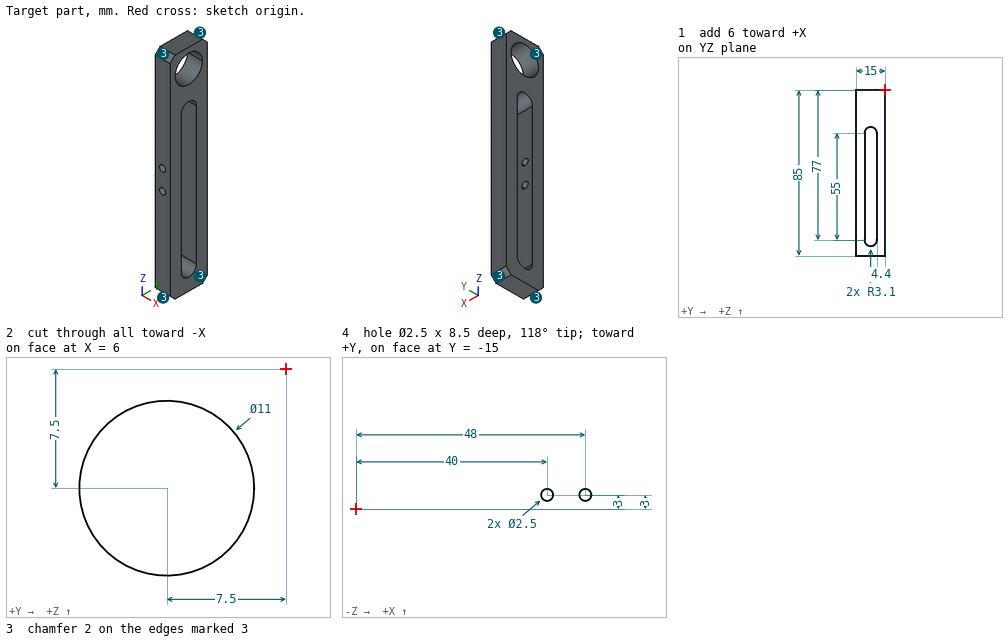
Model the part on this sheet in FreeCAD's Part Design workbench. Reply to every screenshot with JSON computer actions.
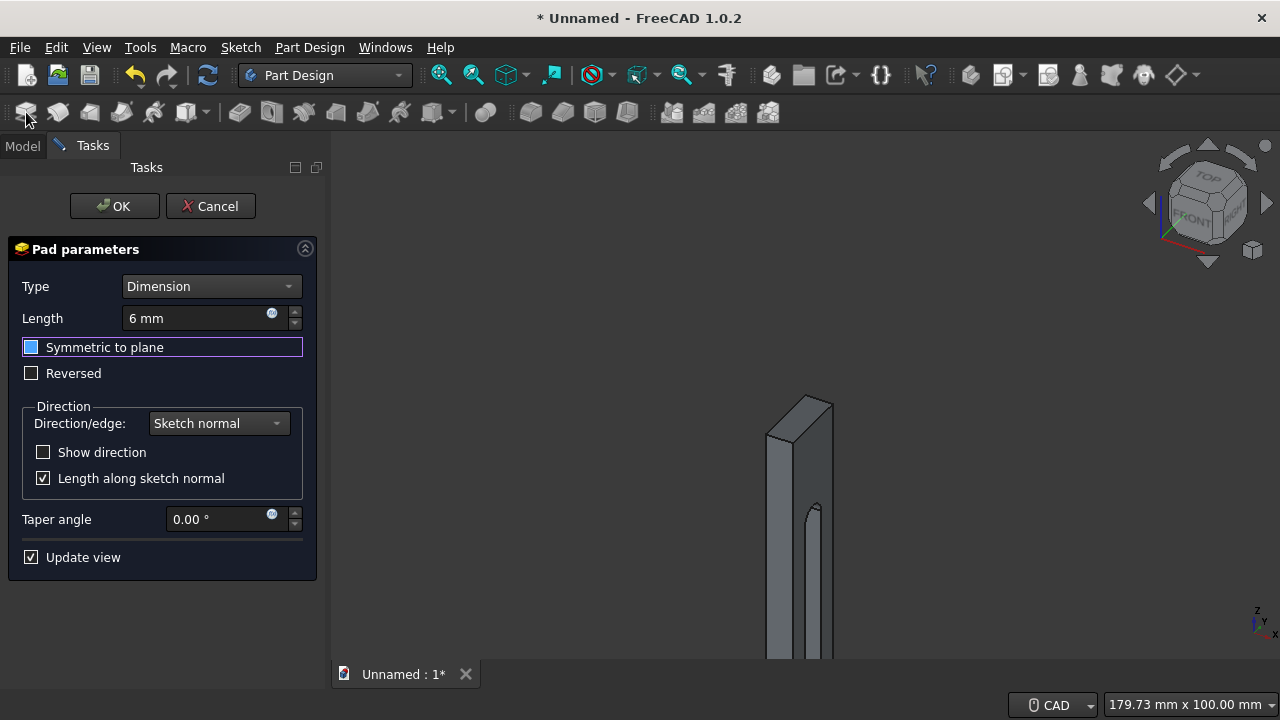
{"action": "left_click", "coordinate": [115, 206]}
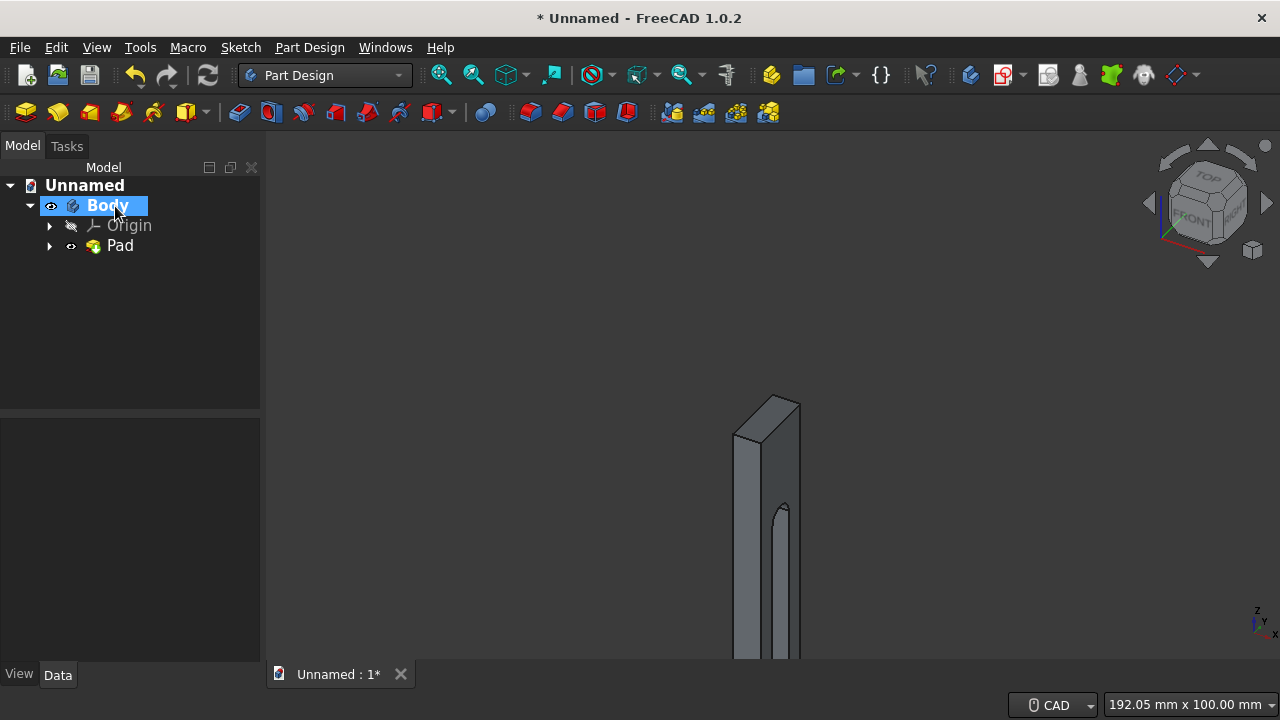
{"action": "key", "text": "v f"}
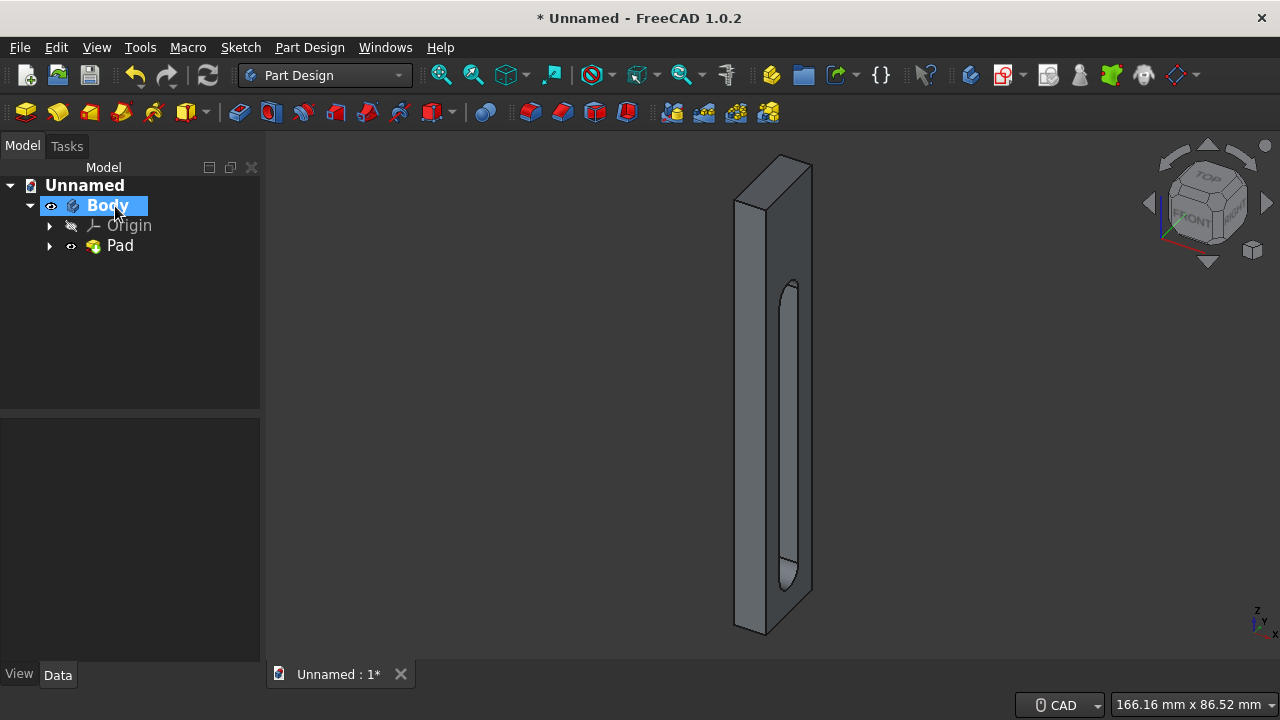
{"action": "left_click", "coordinate": [789, 217]}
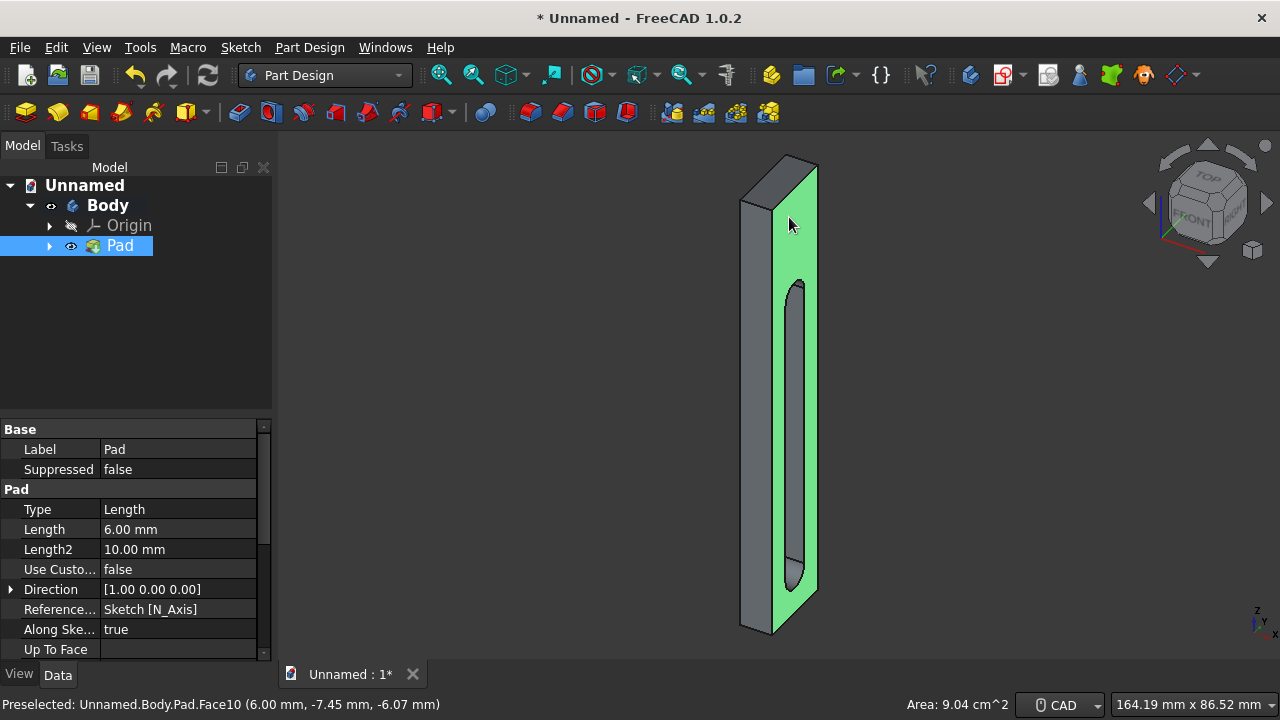
{"action": "left_click", "coordinate": [1004, 76]}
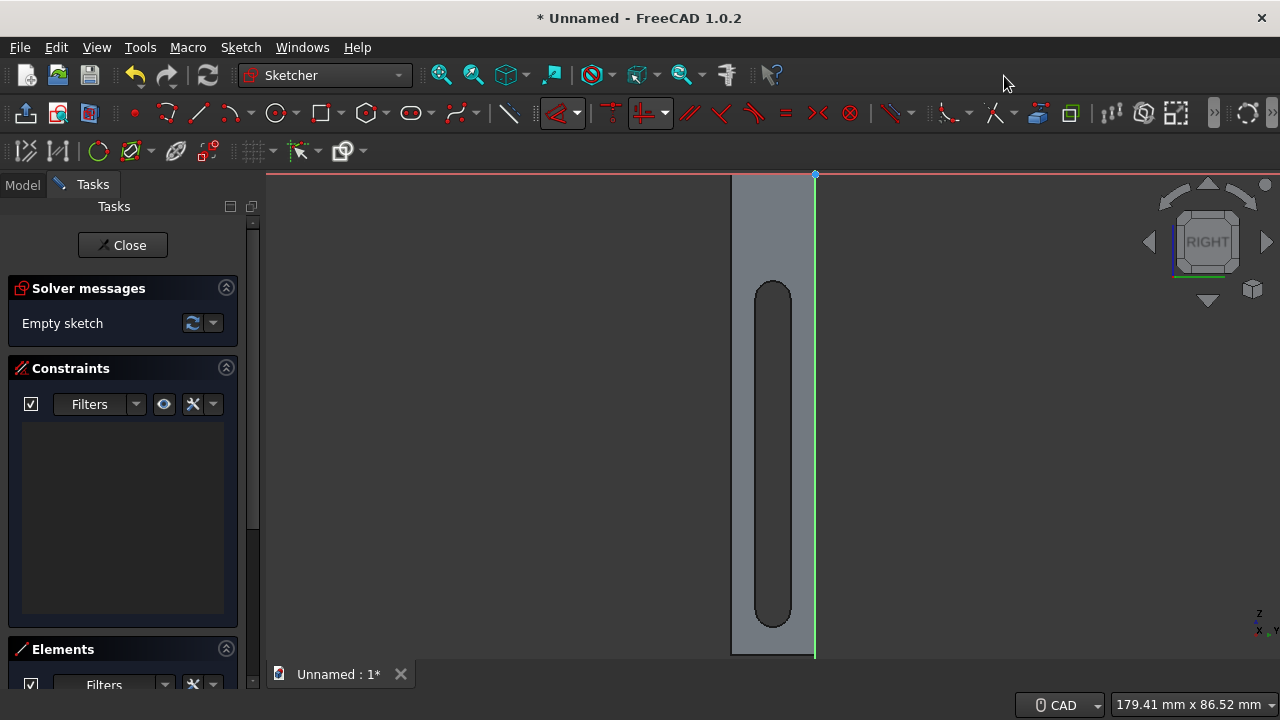
{"action": "scroll", "coordinate": [704, 414], "scroll_direction": "down", "scroll_amount": 5}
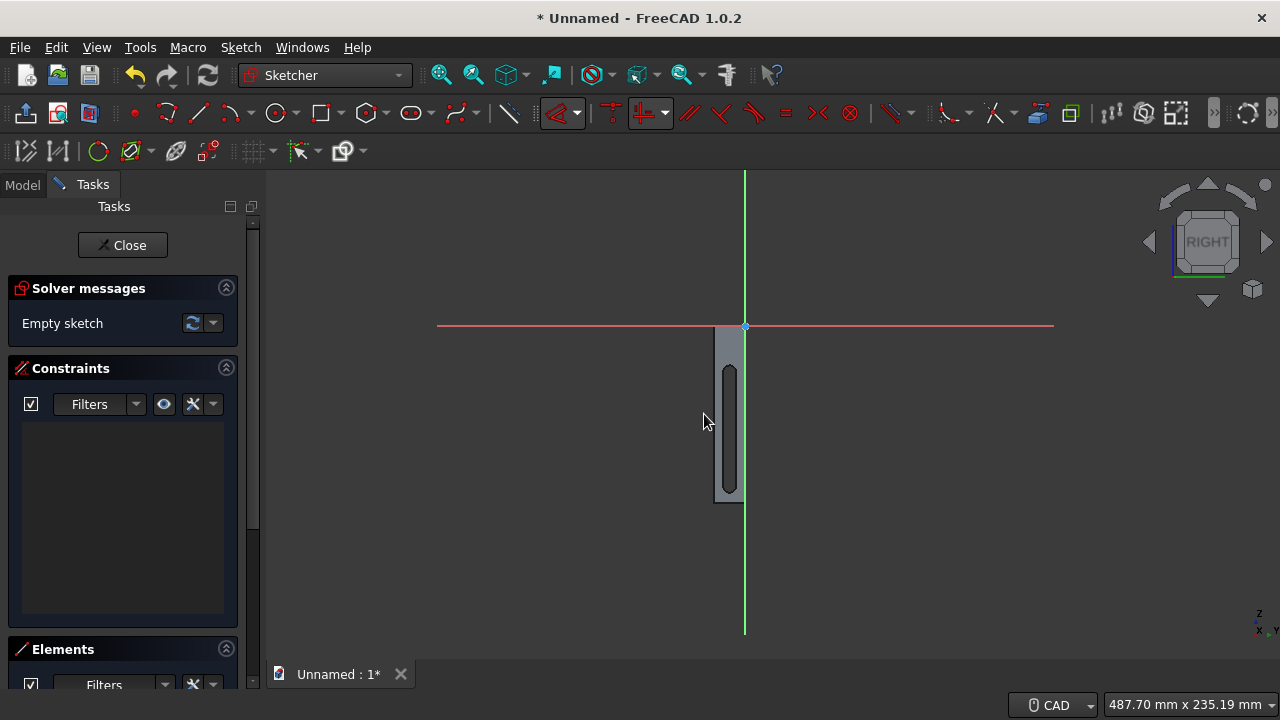
{"action": "scroll", "coordinate": [734, 332], "scroll_direction": "up", "scroll_amount": 12}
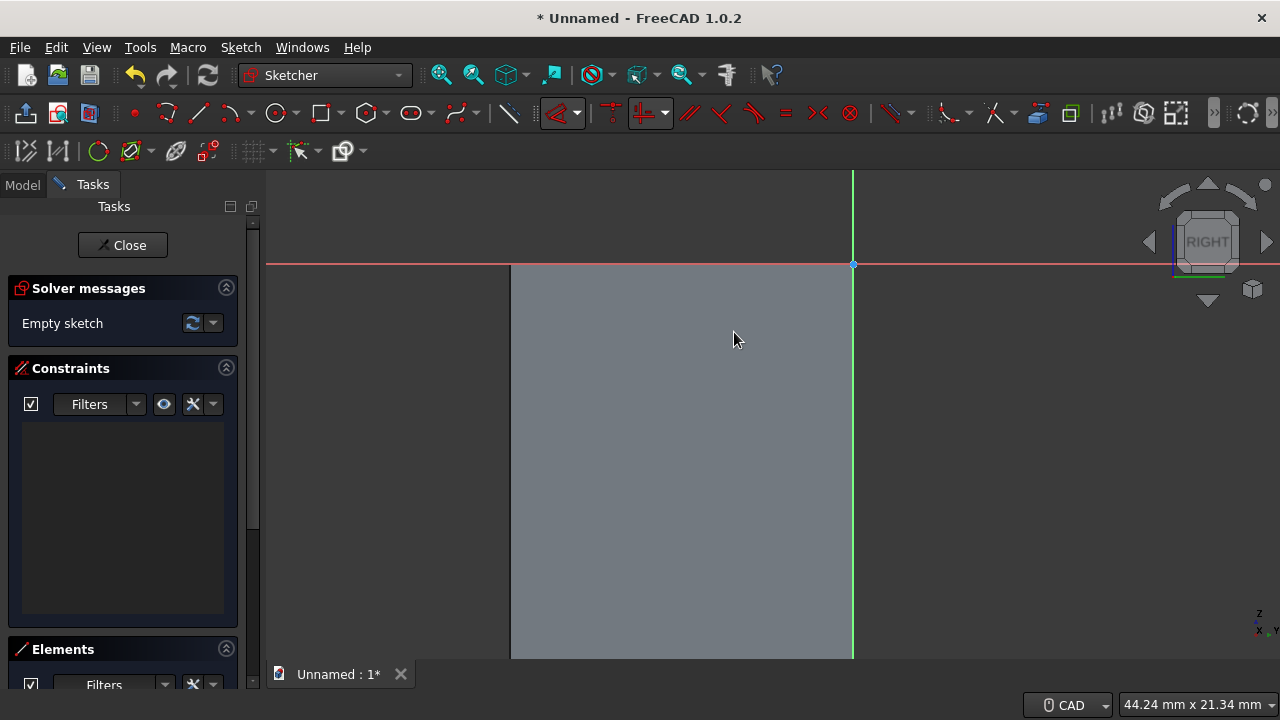
{"action": "key", "text": "g c"}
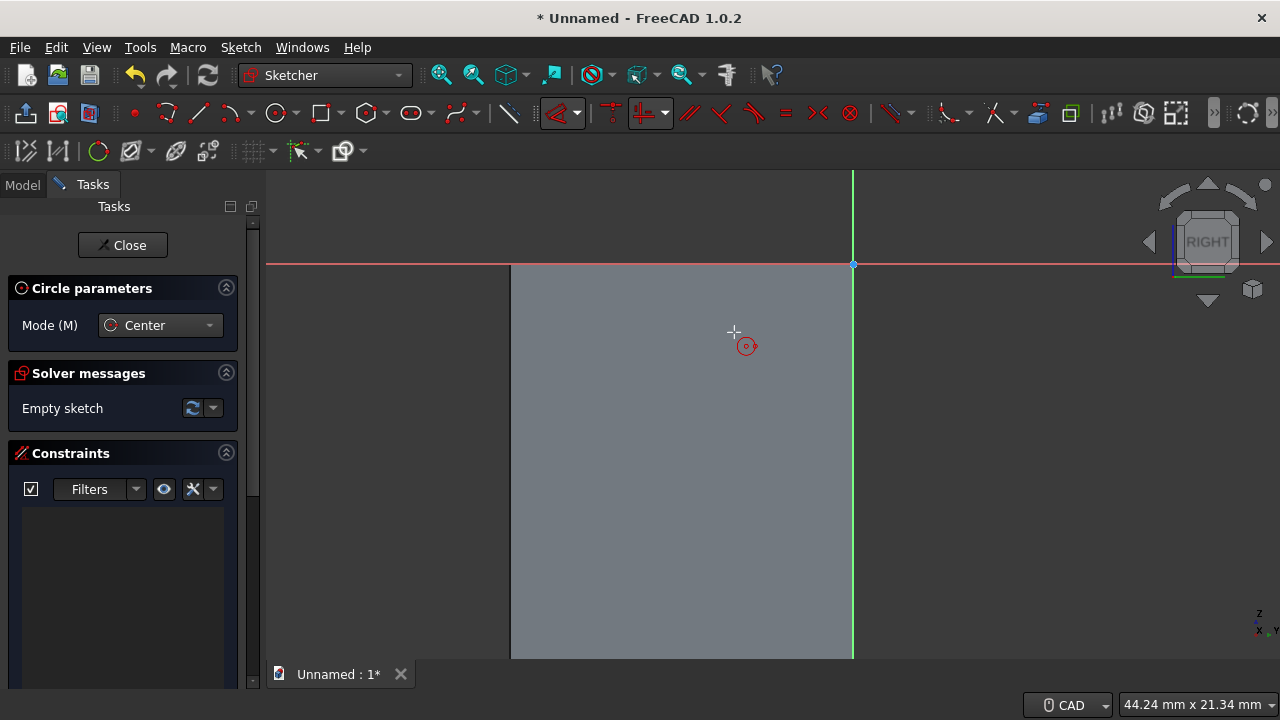
{"action": "left_click", "coordinate": [681, 436]}
{"action": "left_click", "coordinate": [771, 347]}
{"action": "key", "text": "Escape"}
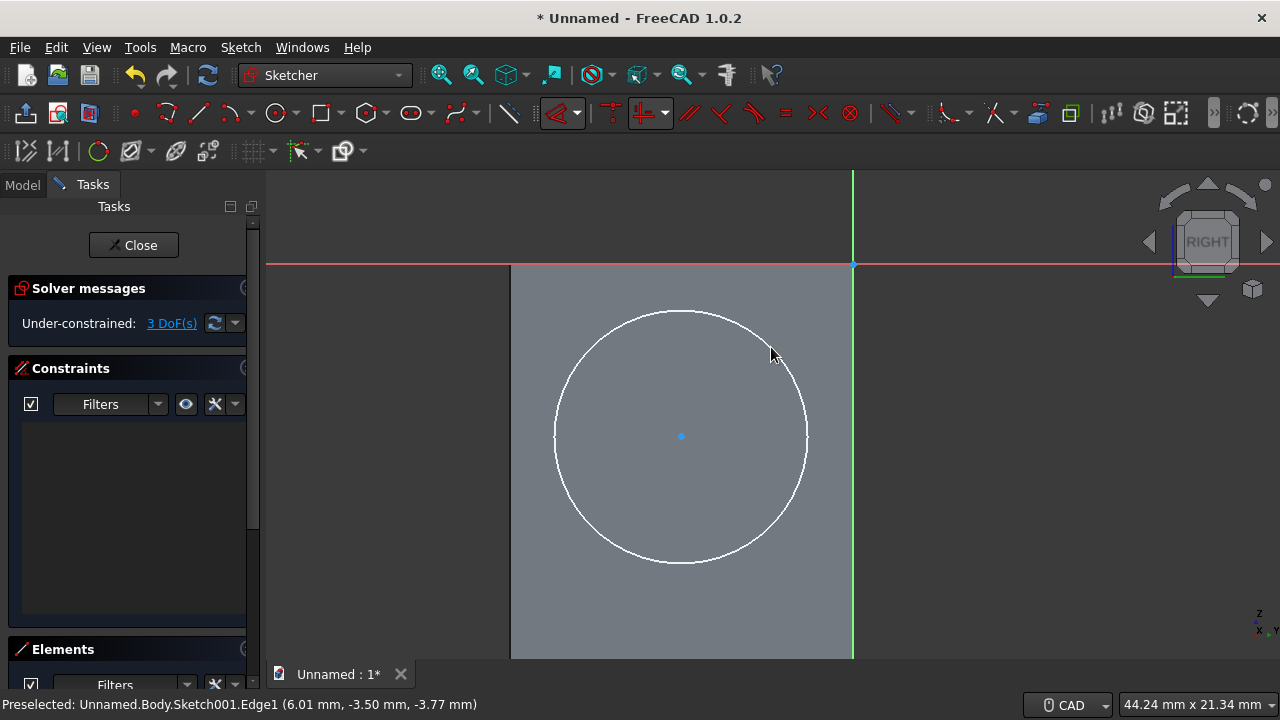
{"action": "key", "text": "d"}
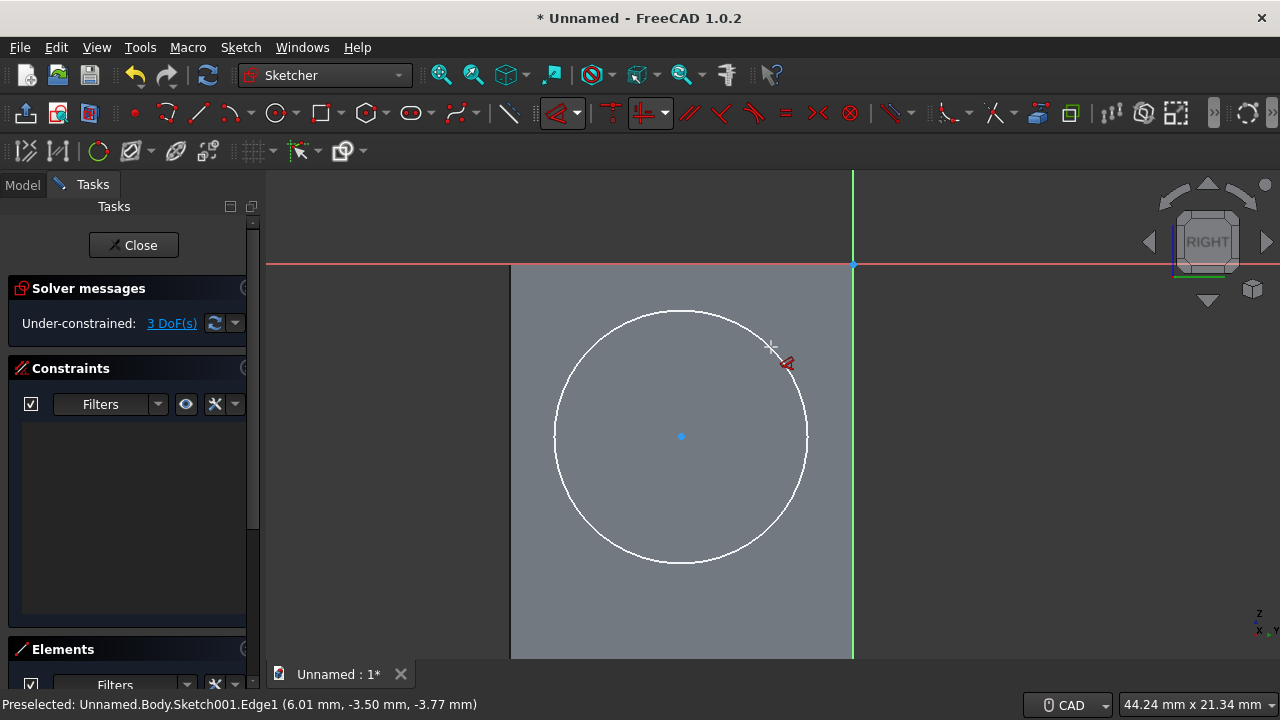
{"action": "left_click", "coordinate": [770, 347]}
{"action": "left_click", "coordinate": [793, 324]}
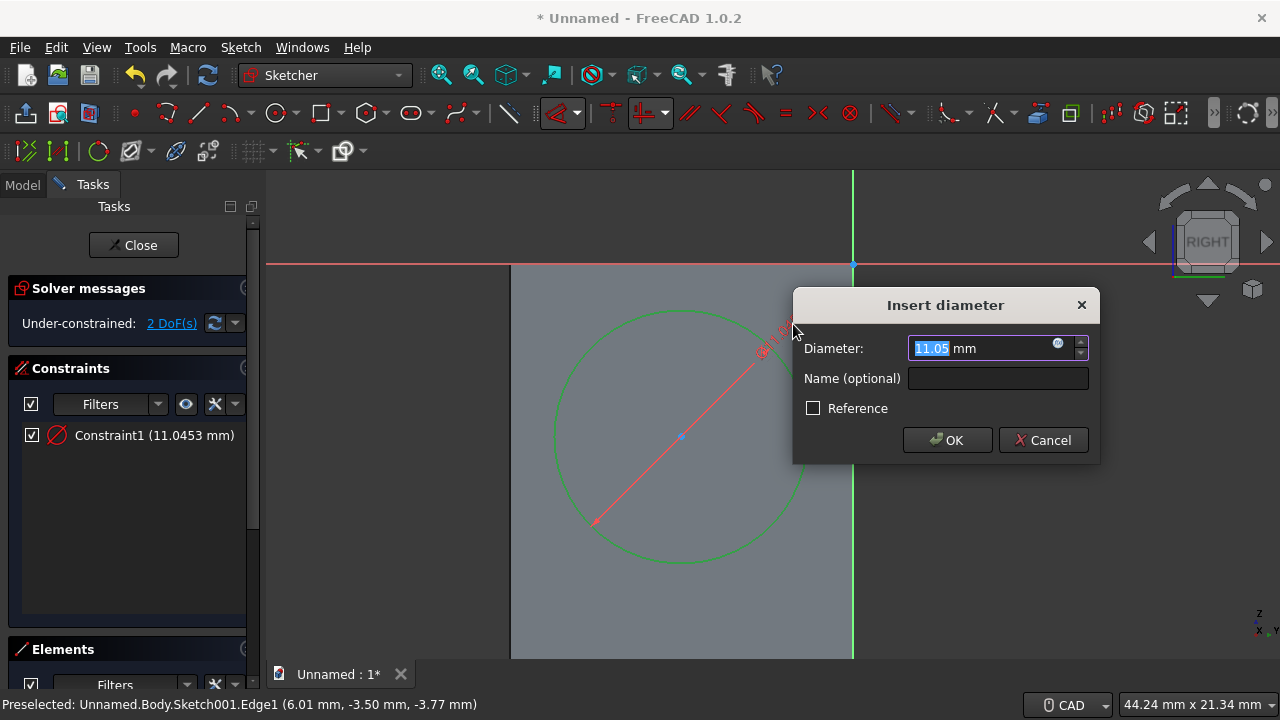
{"action": "type", "text": "11"}
{"action": "key", "text": "Return"}